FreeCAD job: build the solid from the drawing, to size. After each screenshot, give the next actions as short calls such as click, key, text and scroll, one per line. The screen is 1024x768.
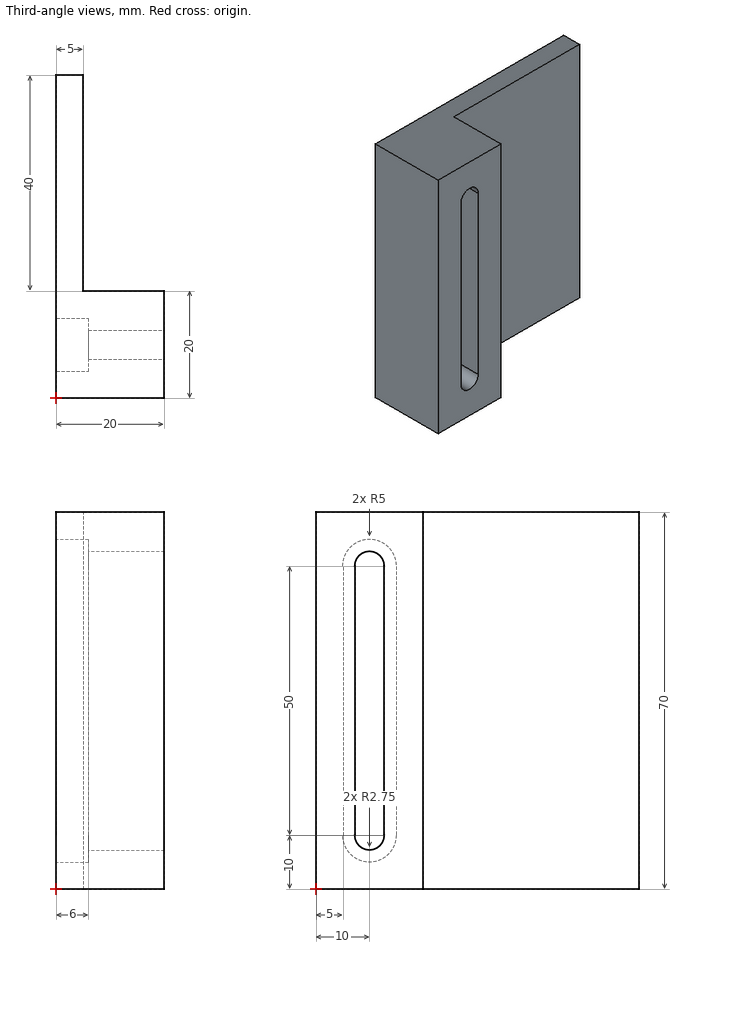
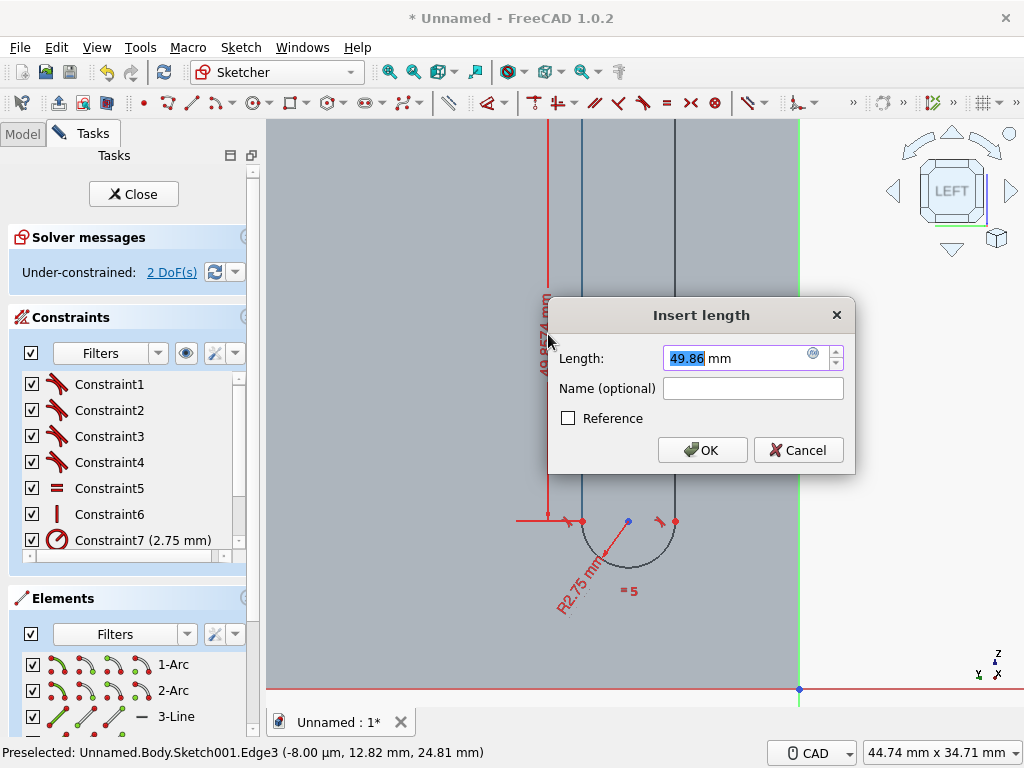
text(50)
key(Return)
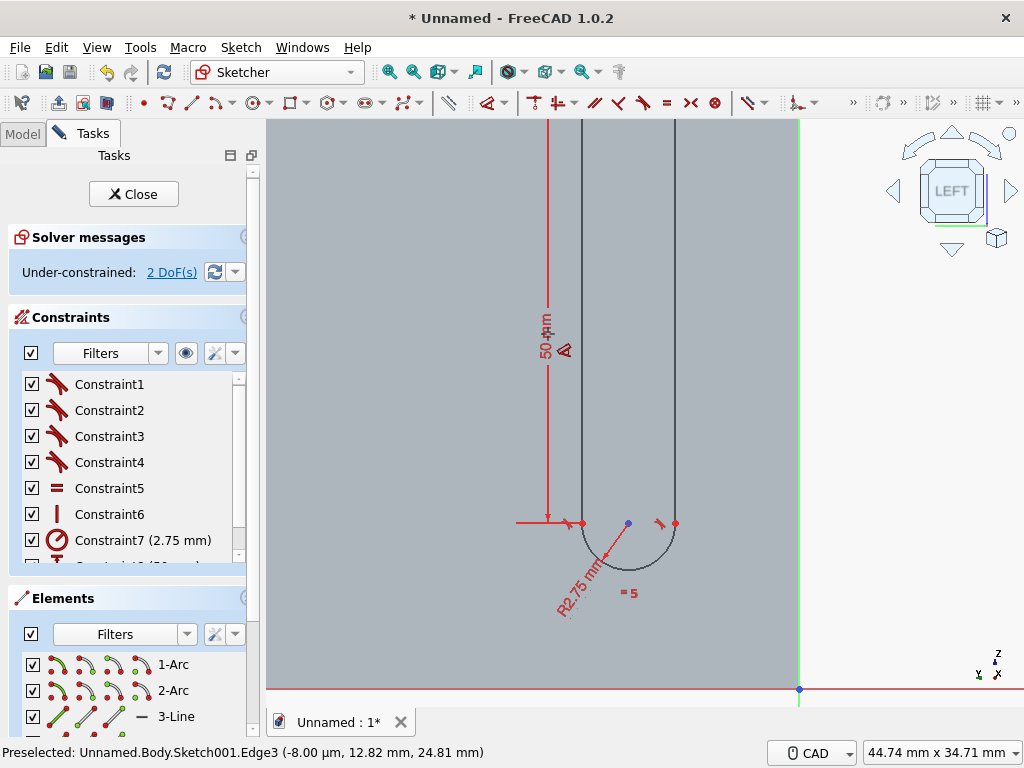
click(582, 523)
click(548, 637)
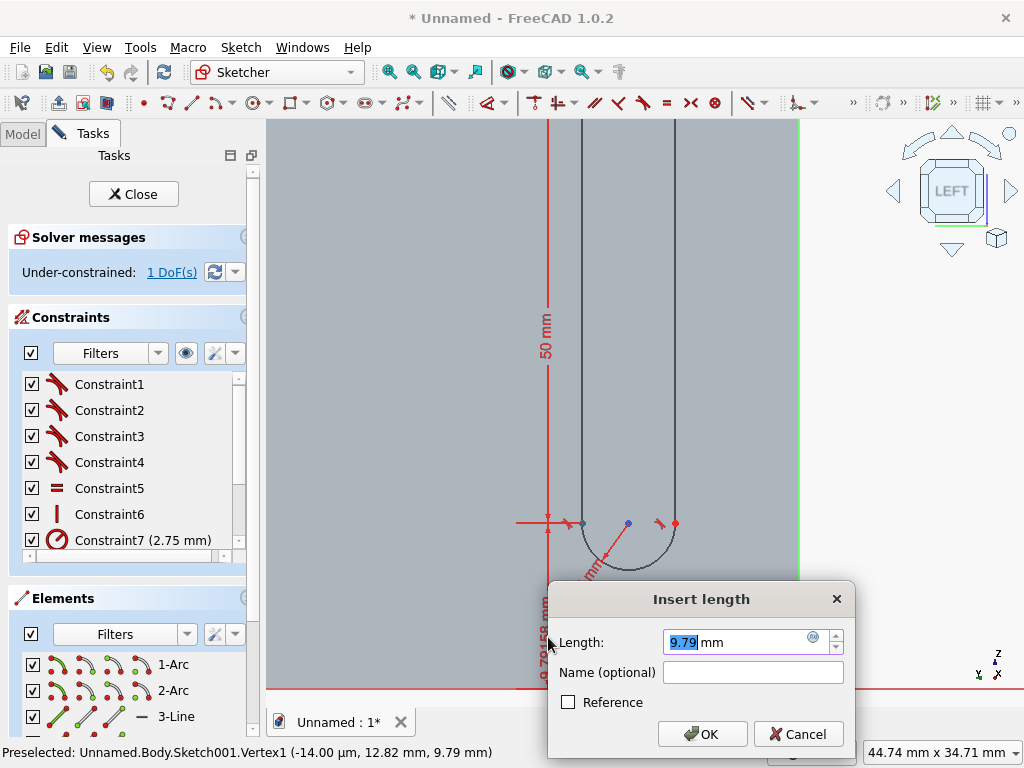
text(10)
key(Return)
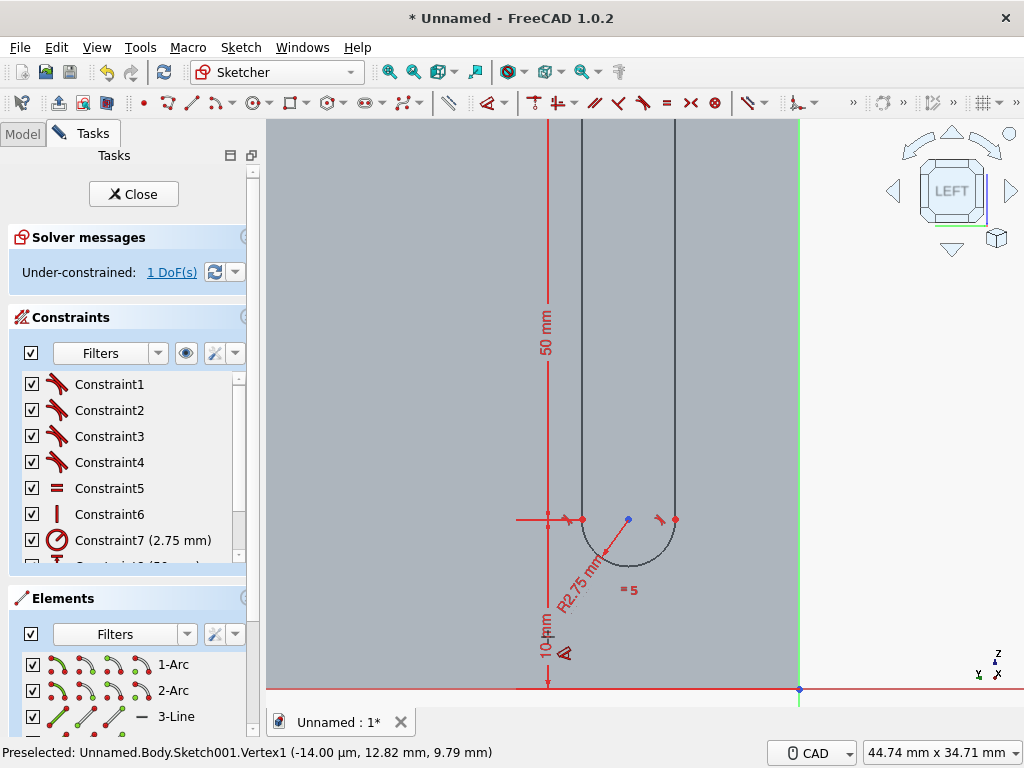
click(629, 520)
click(714, 486)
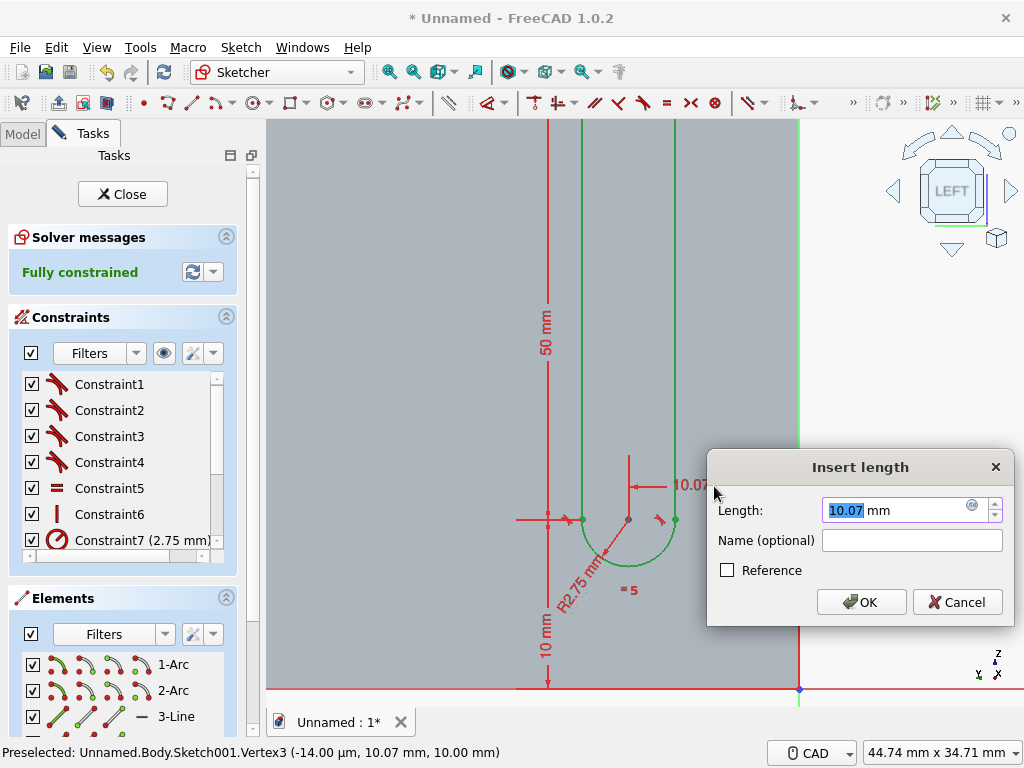
text(10)
key(Return)
key(Escape)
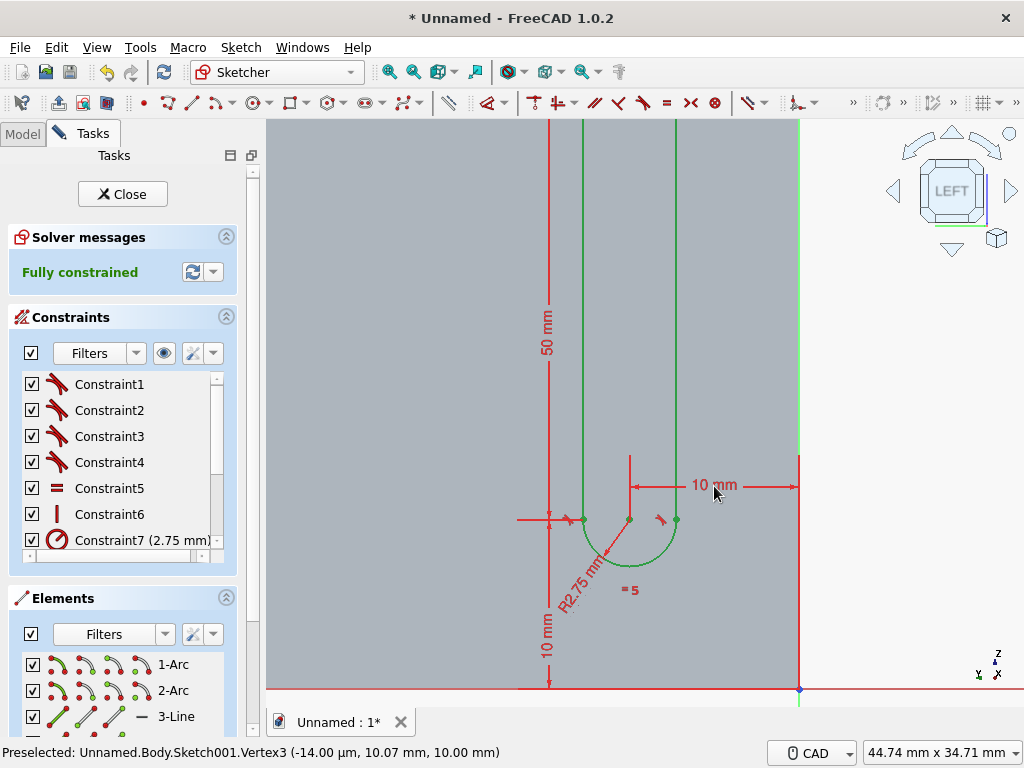
click(123, 194)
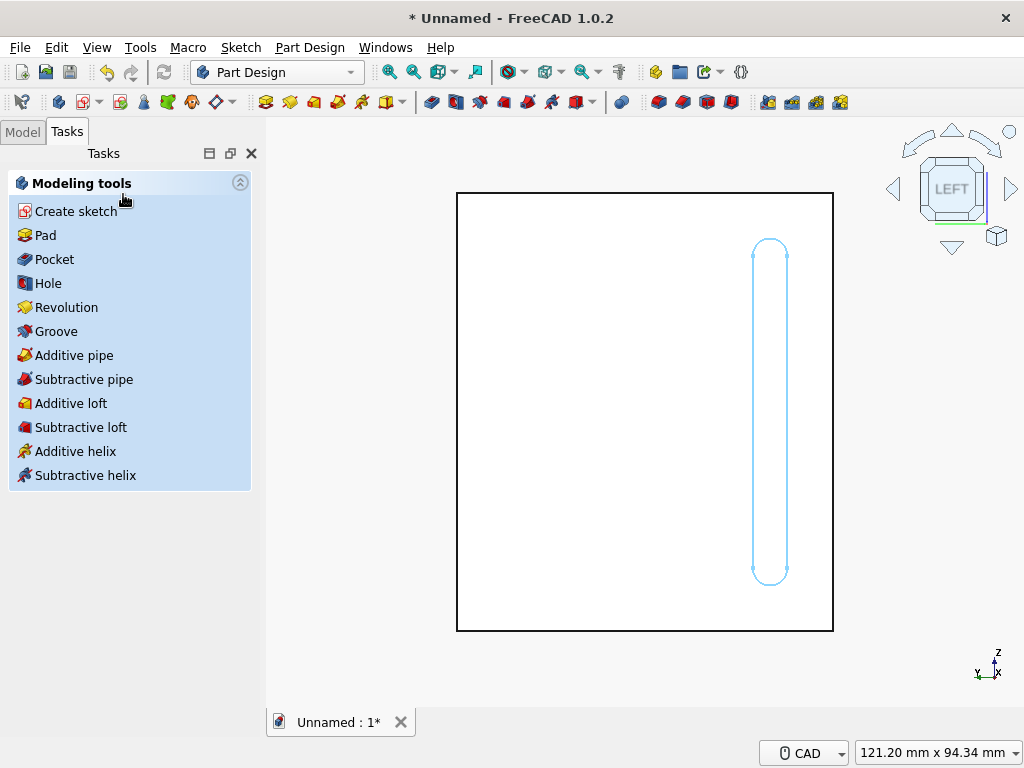
click(432, 102)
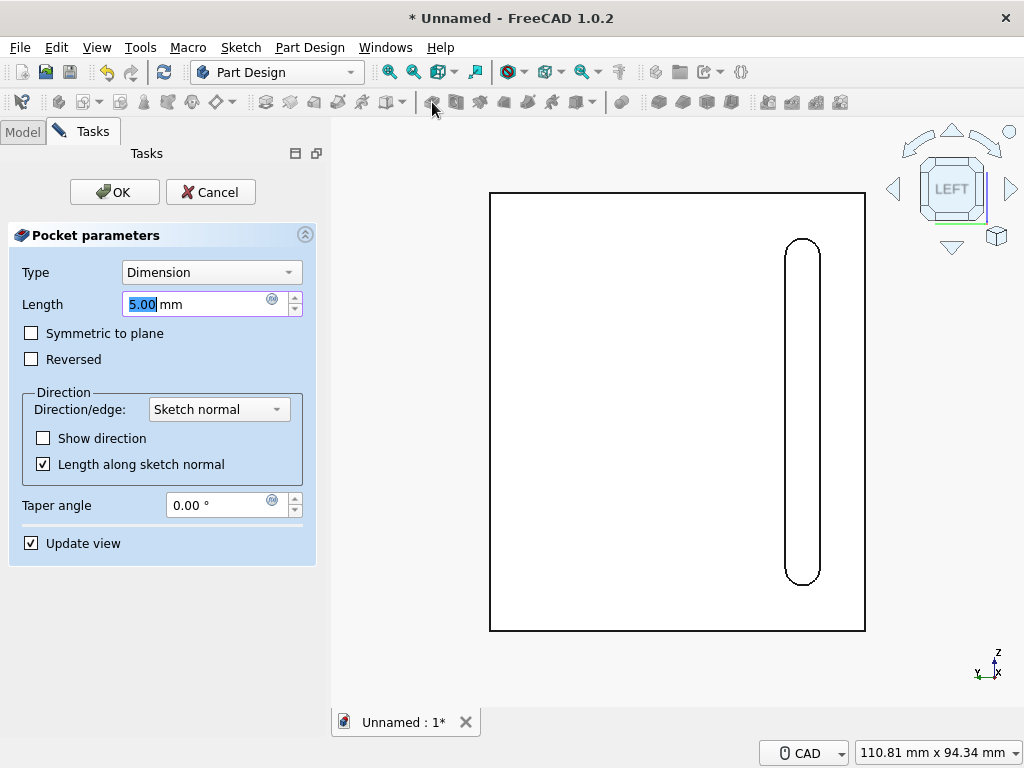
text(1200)
key(Tab)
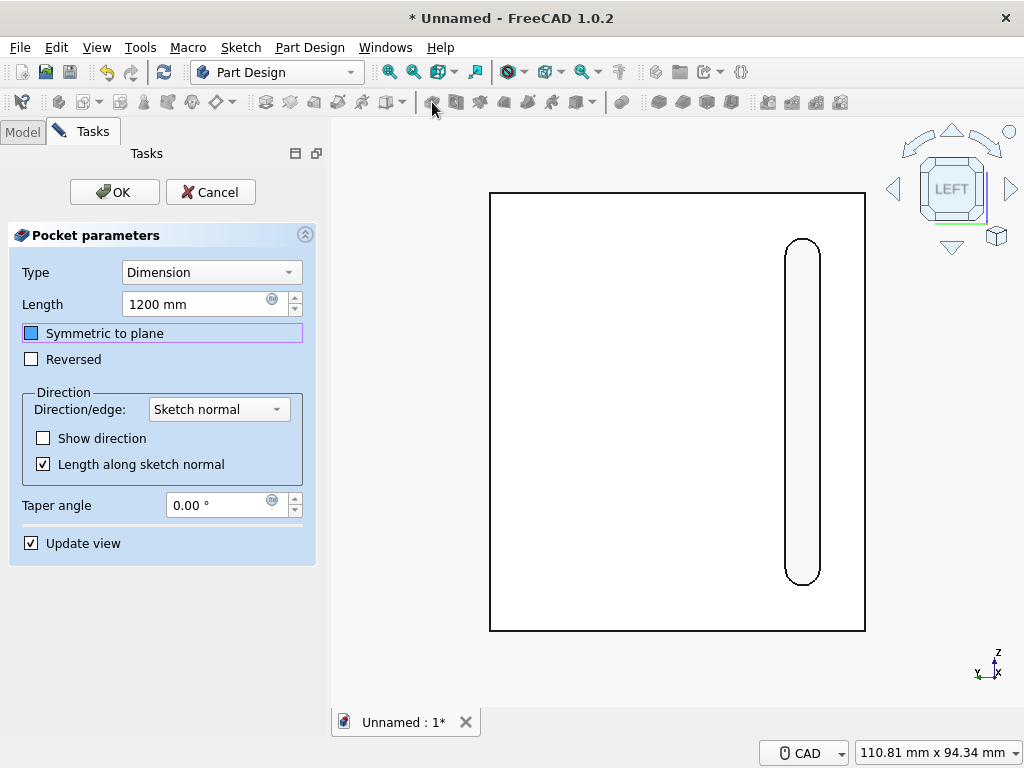
click(115, 192)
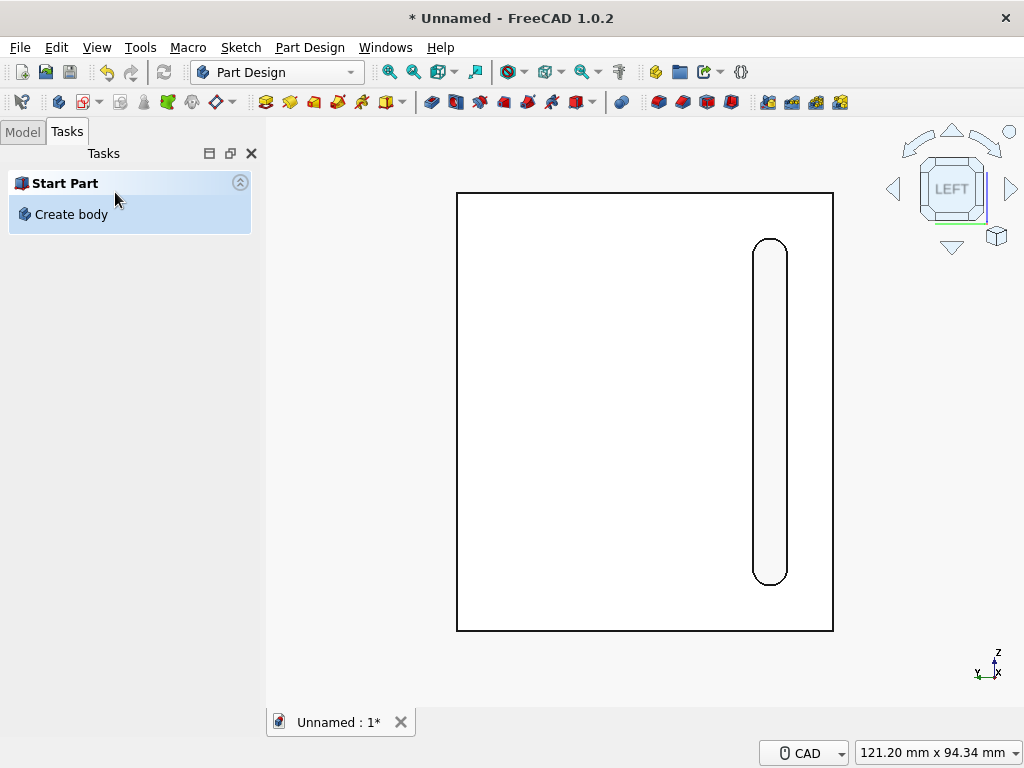
click(591, 348)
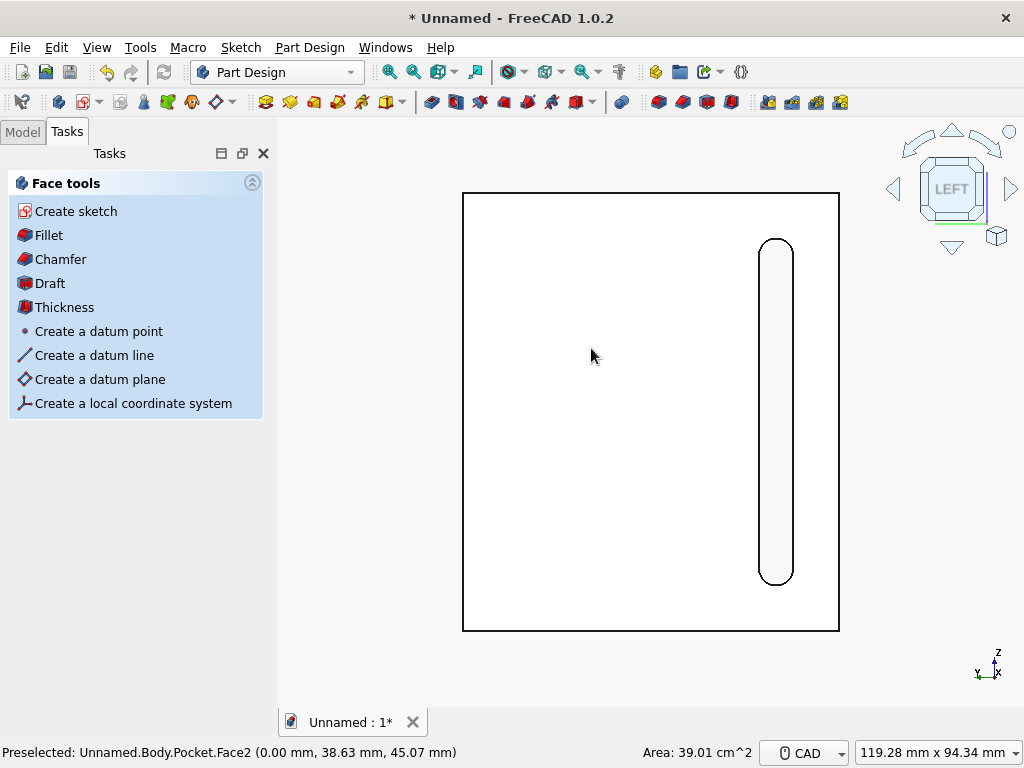
click(84, 102)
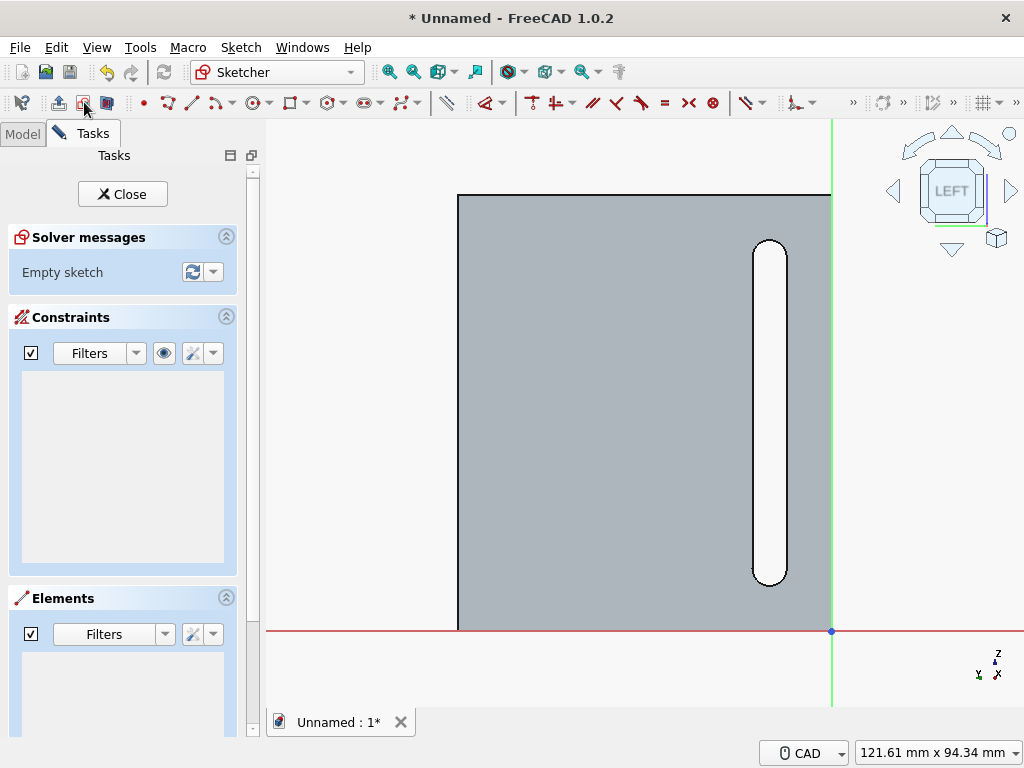
click(364, 104)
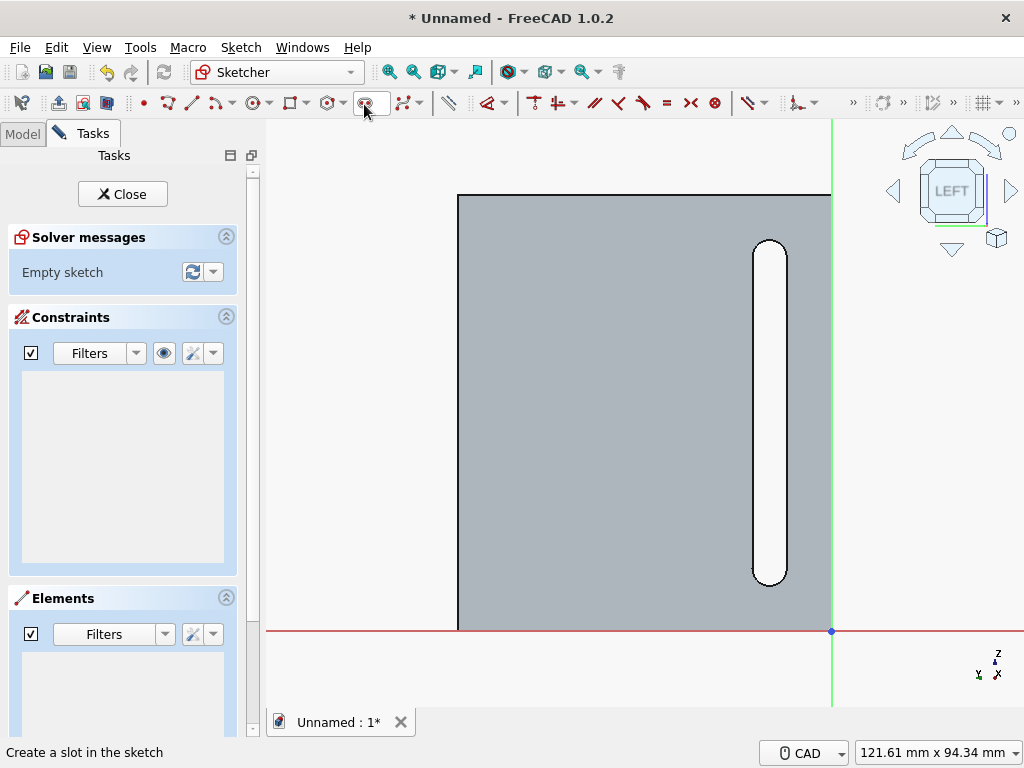
click(770, 569)